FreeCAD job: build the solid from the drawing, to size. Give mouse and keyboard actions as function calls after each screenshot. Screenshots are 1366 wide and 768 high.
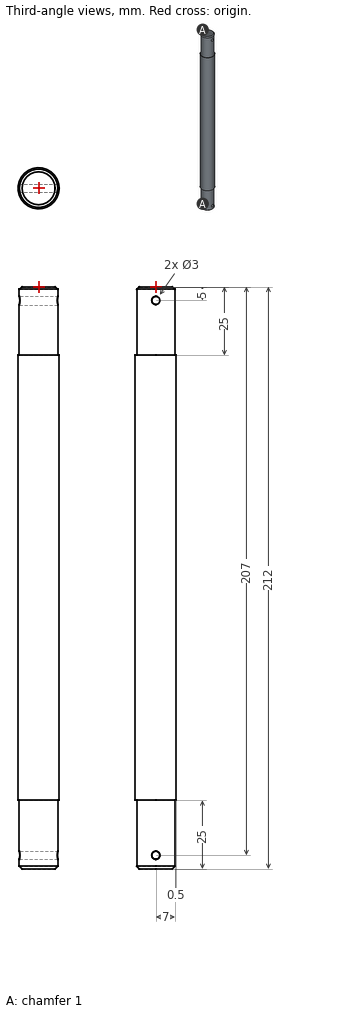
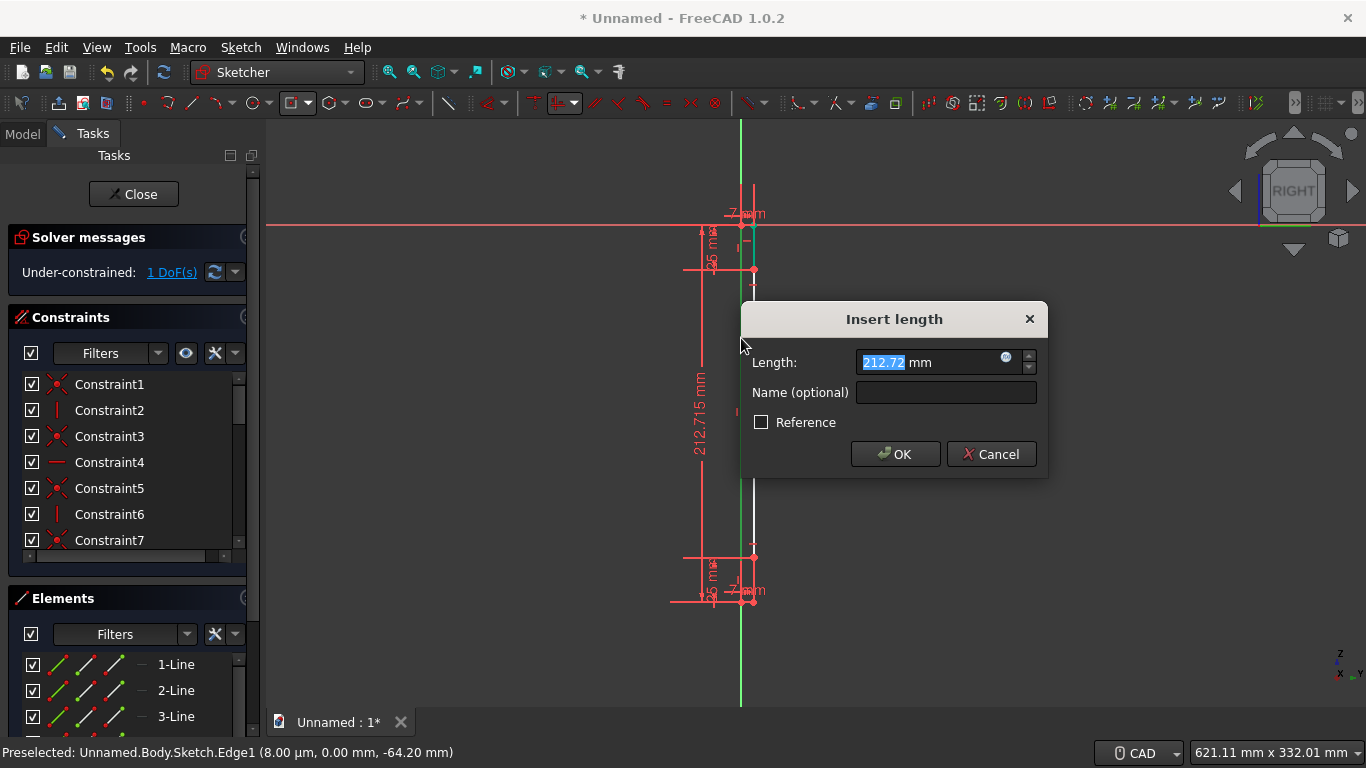
text(212)
key(Return)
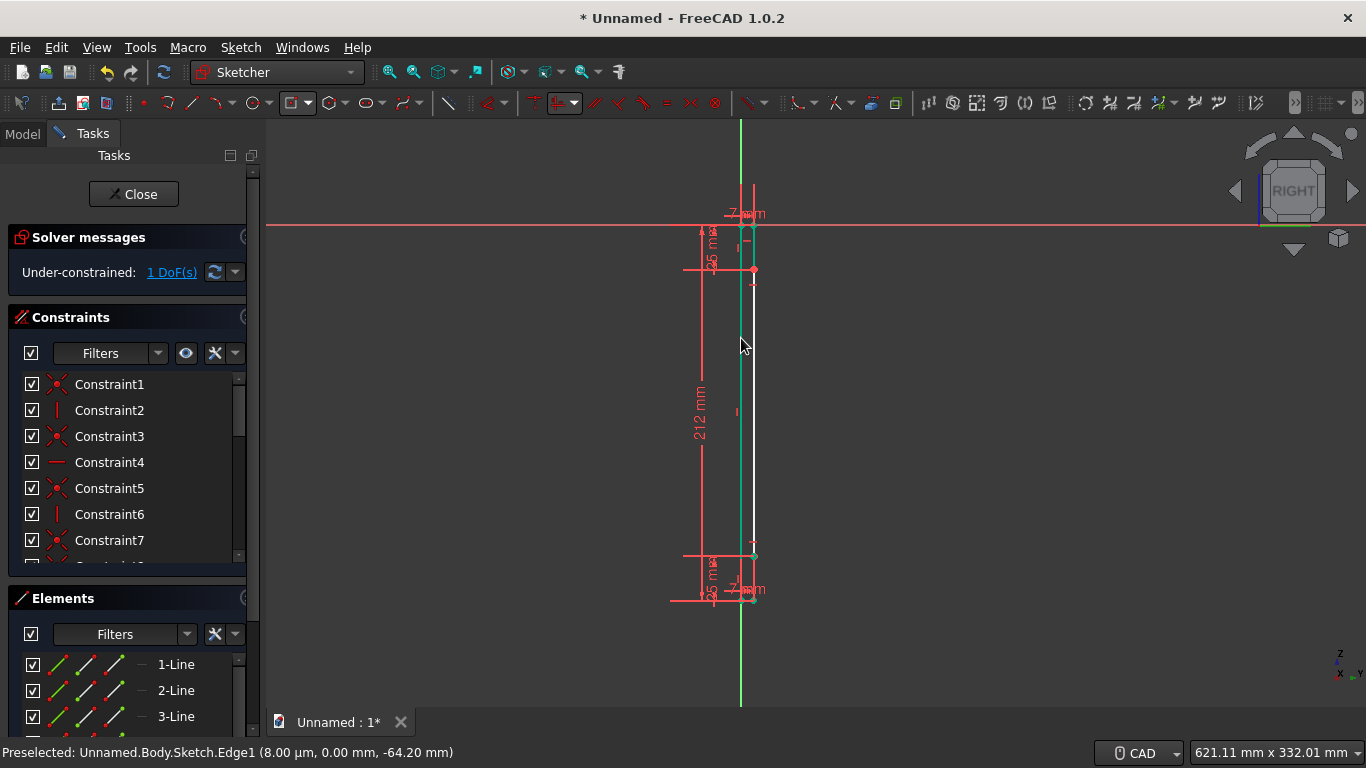
scroll(754, 556, up, 20)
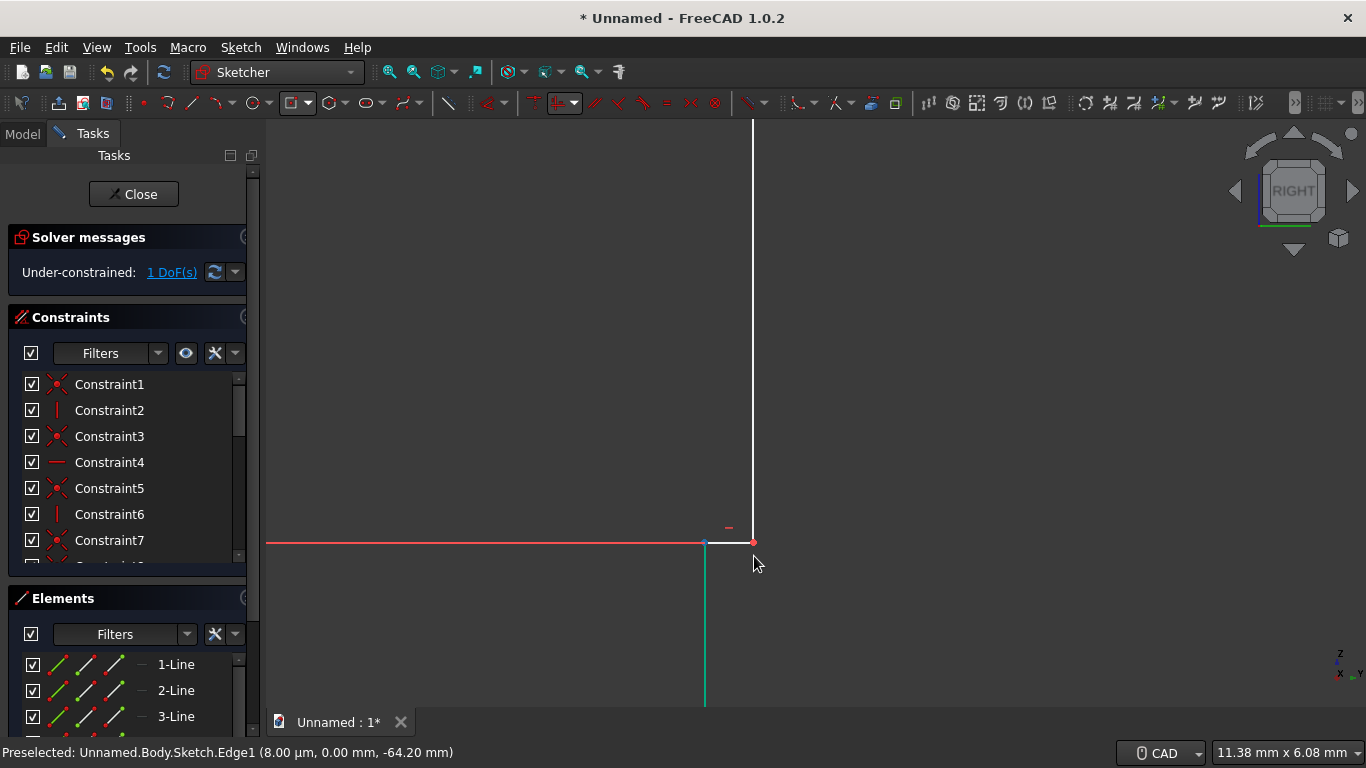
click(729, 543)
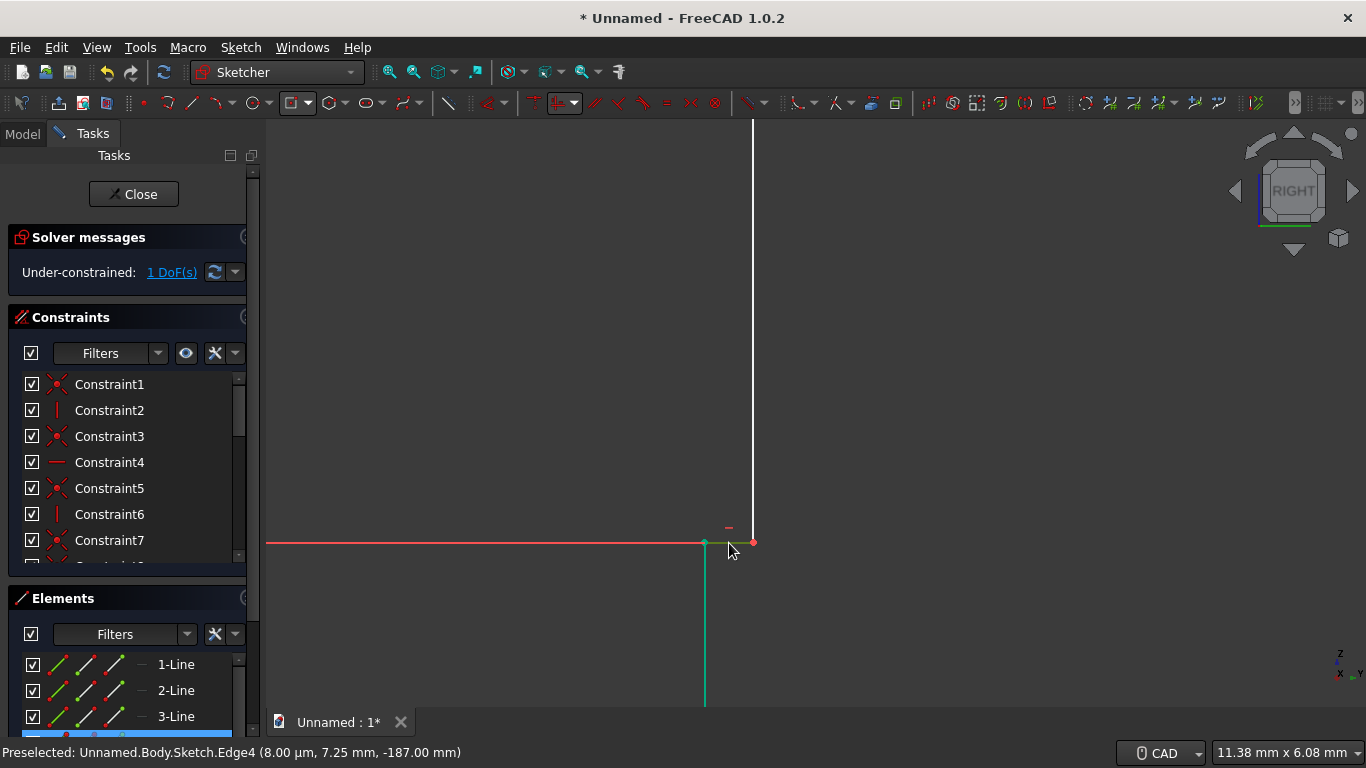
key(l)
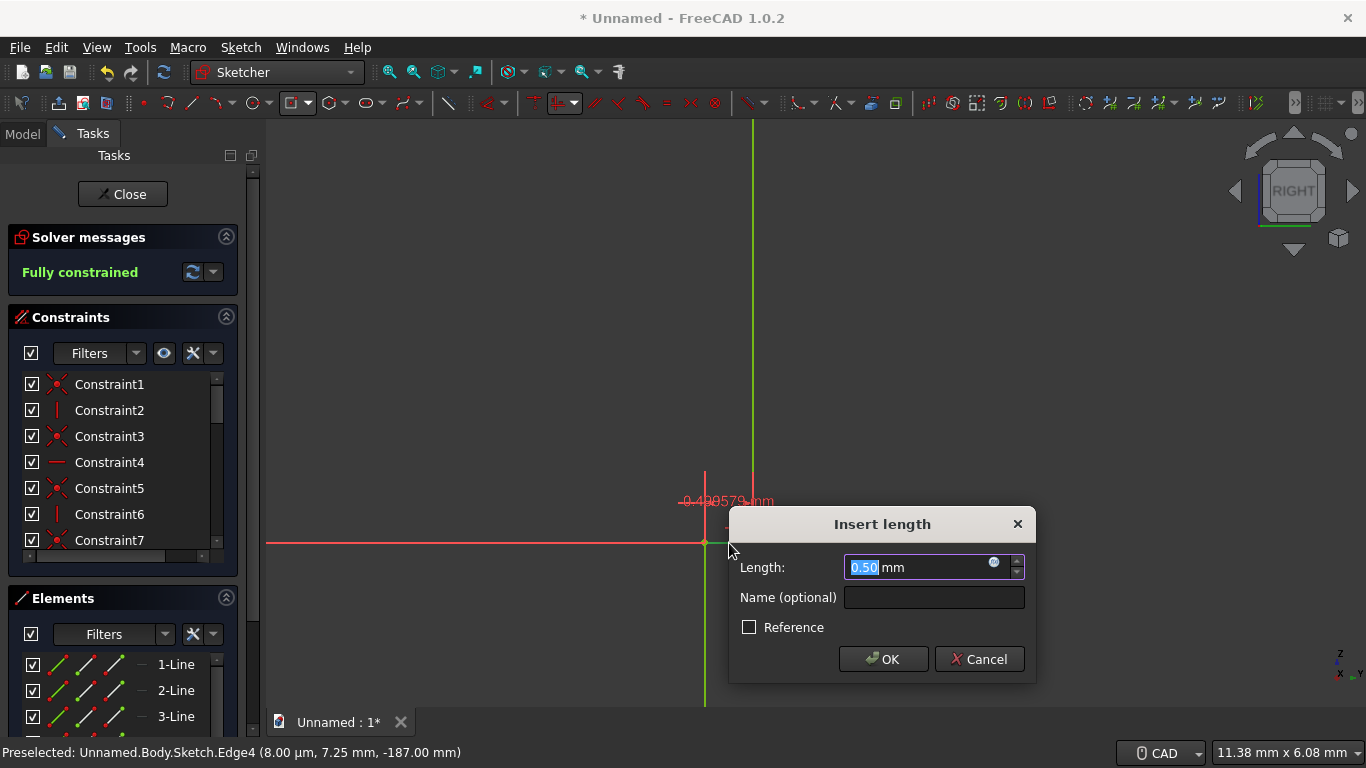
text(0.5)
key(Return)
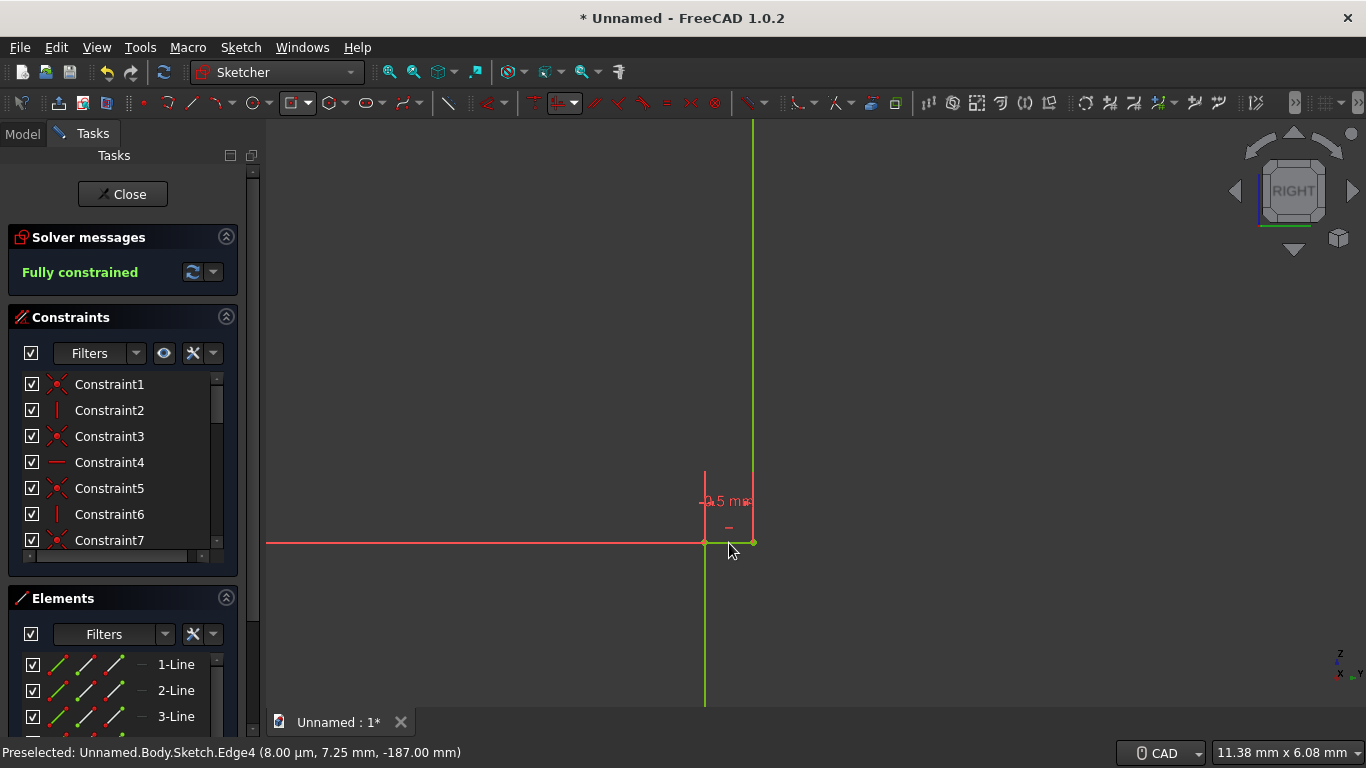
click(123, 194)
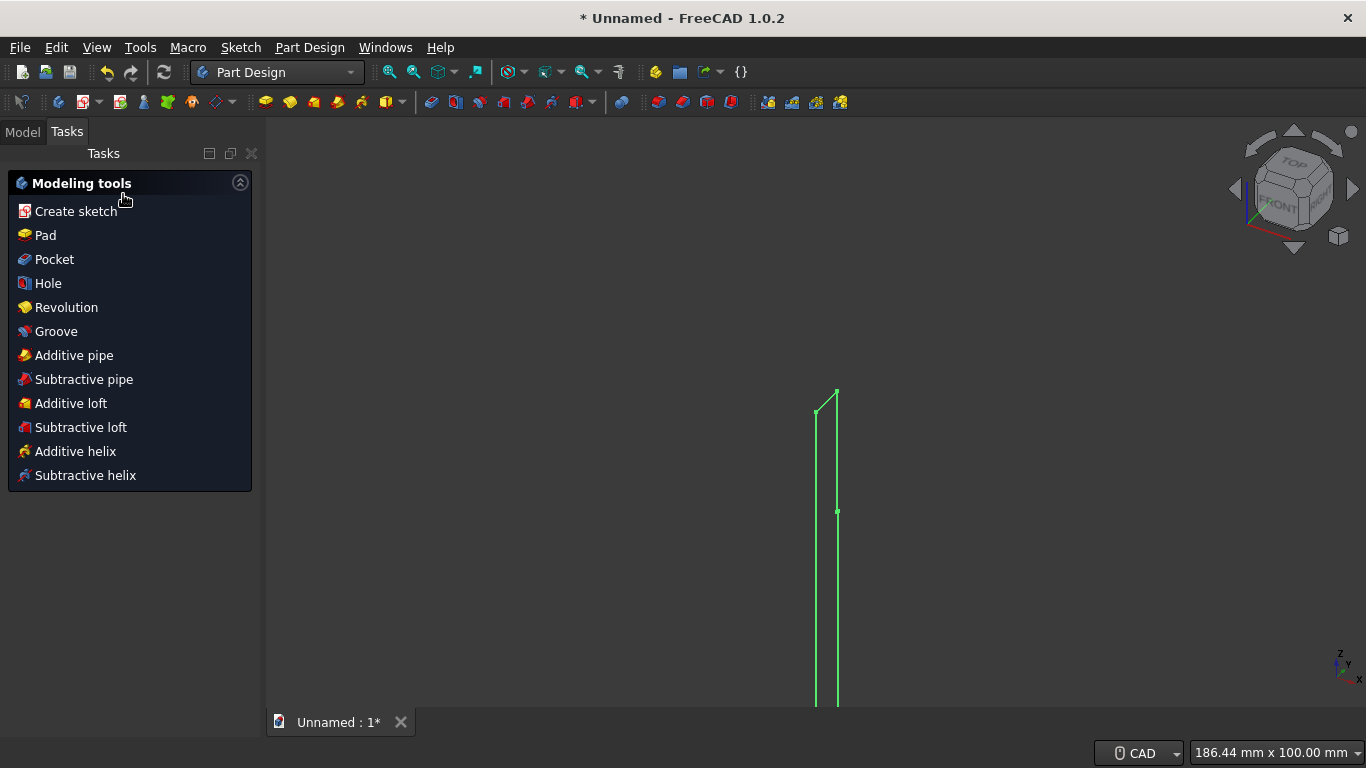
click(290, 102)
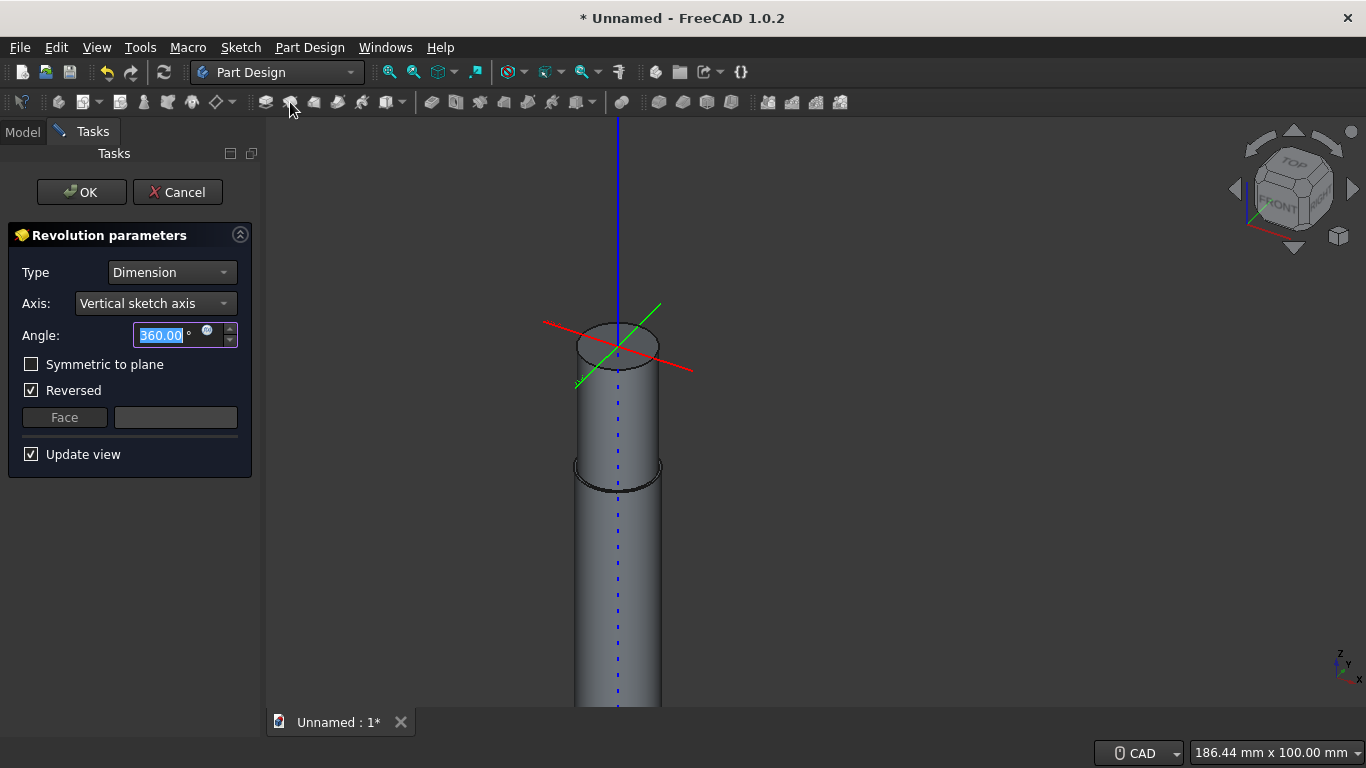
click(82, 192)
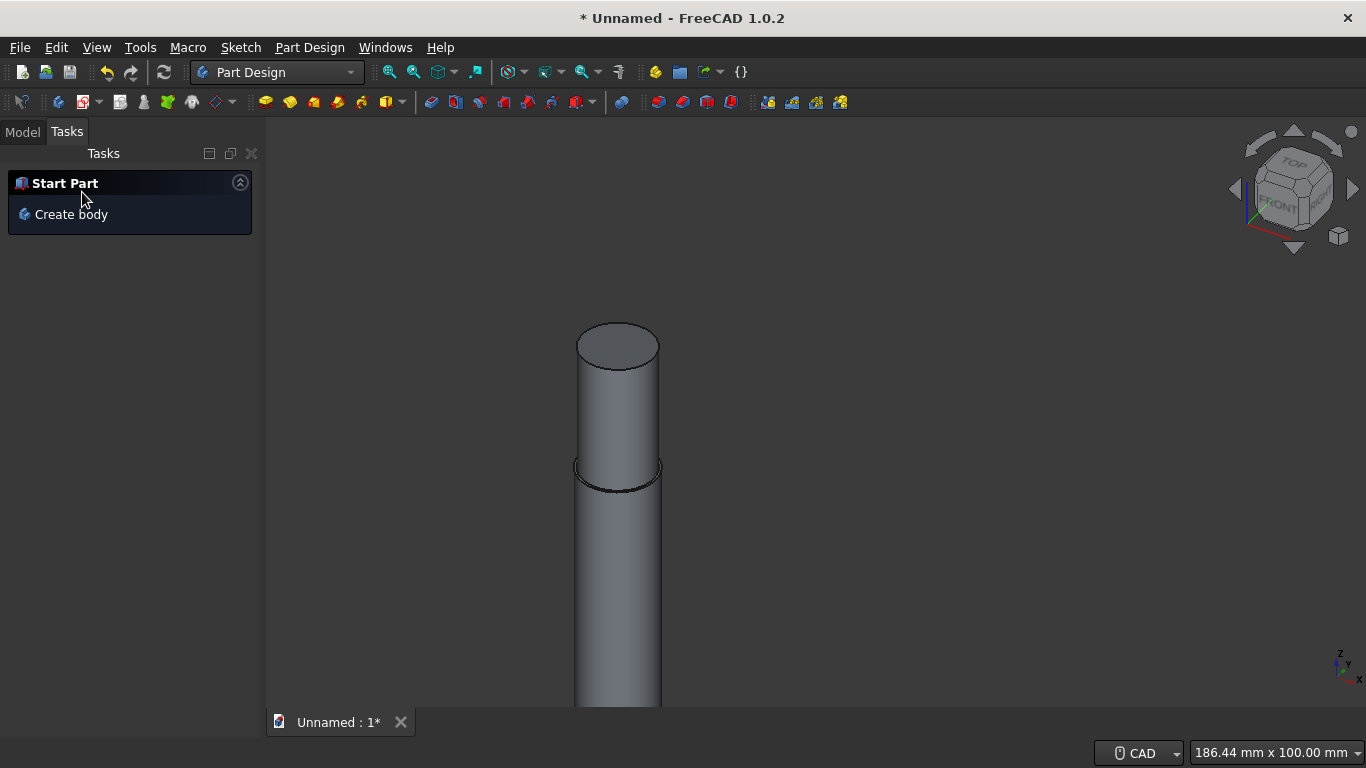
key(v)
key(f)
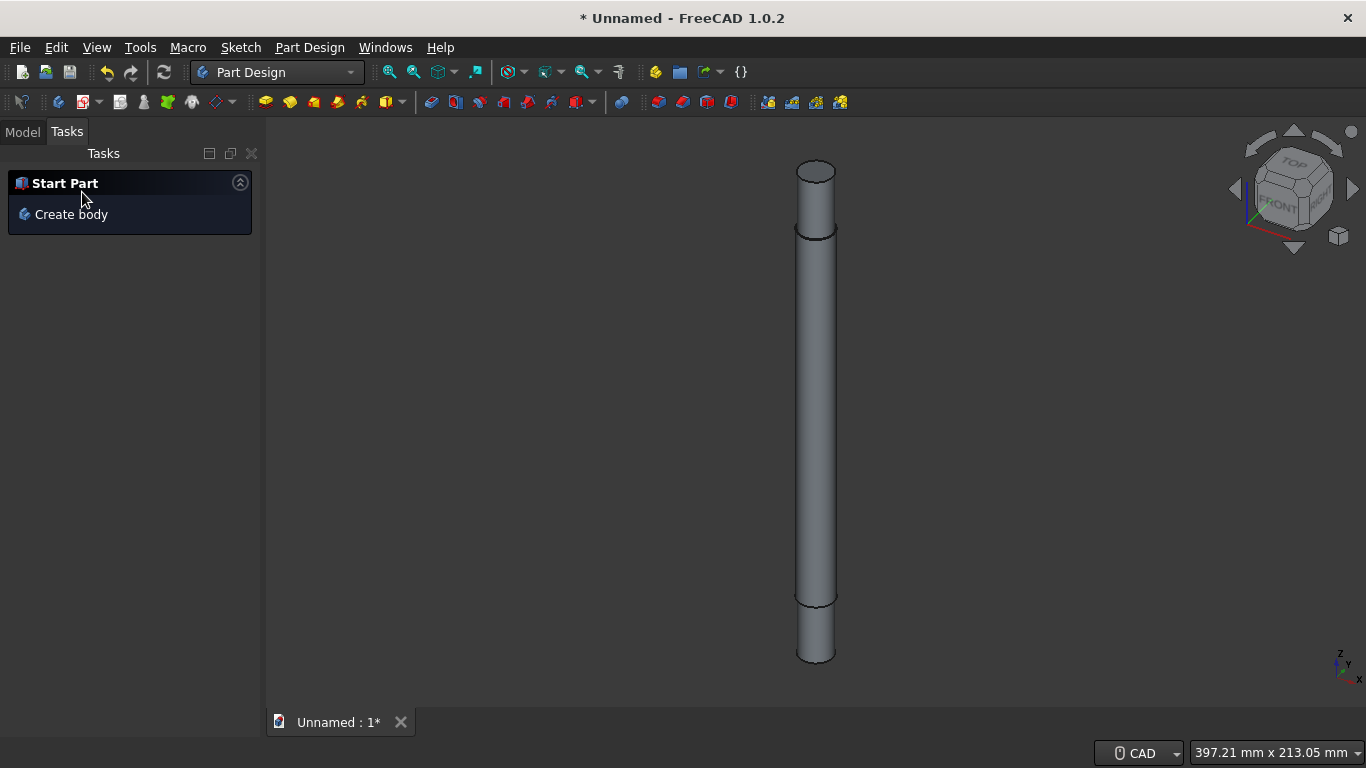
click(84, 102)